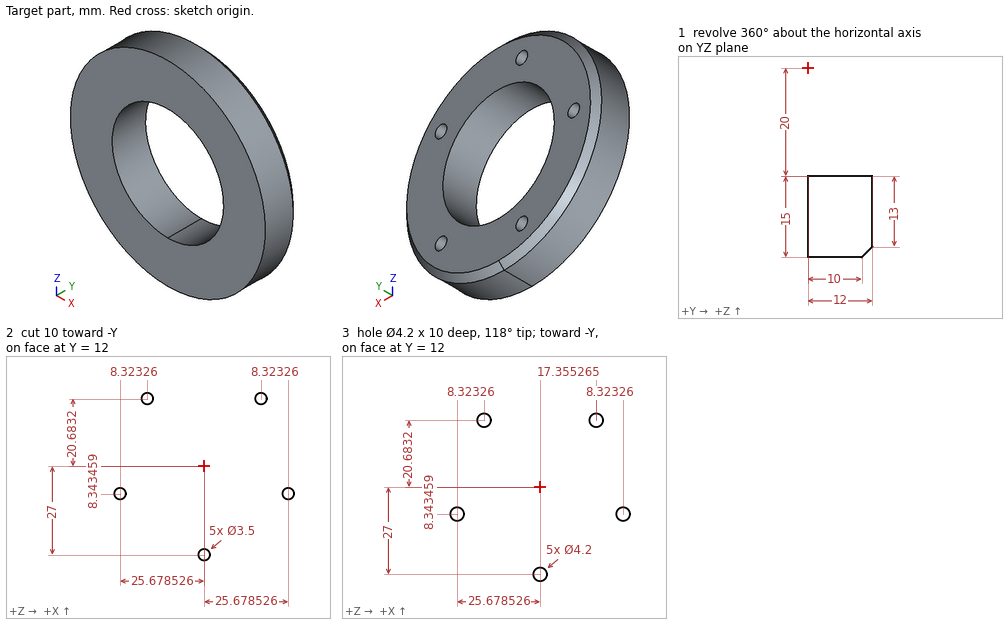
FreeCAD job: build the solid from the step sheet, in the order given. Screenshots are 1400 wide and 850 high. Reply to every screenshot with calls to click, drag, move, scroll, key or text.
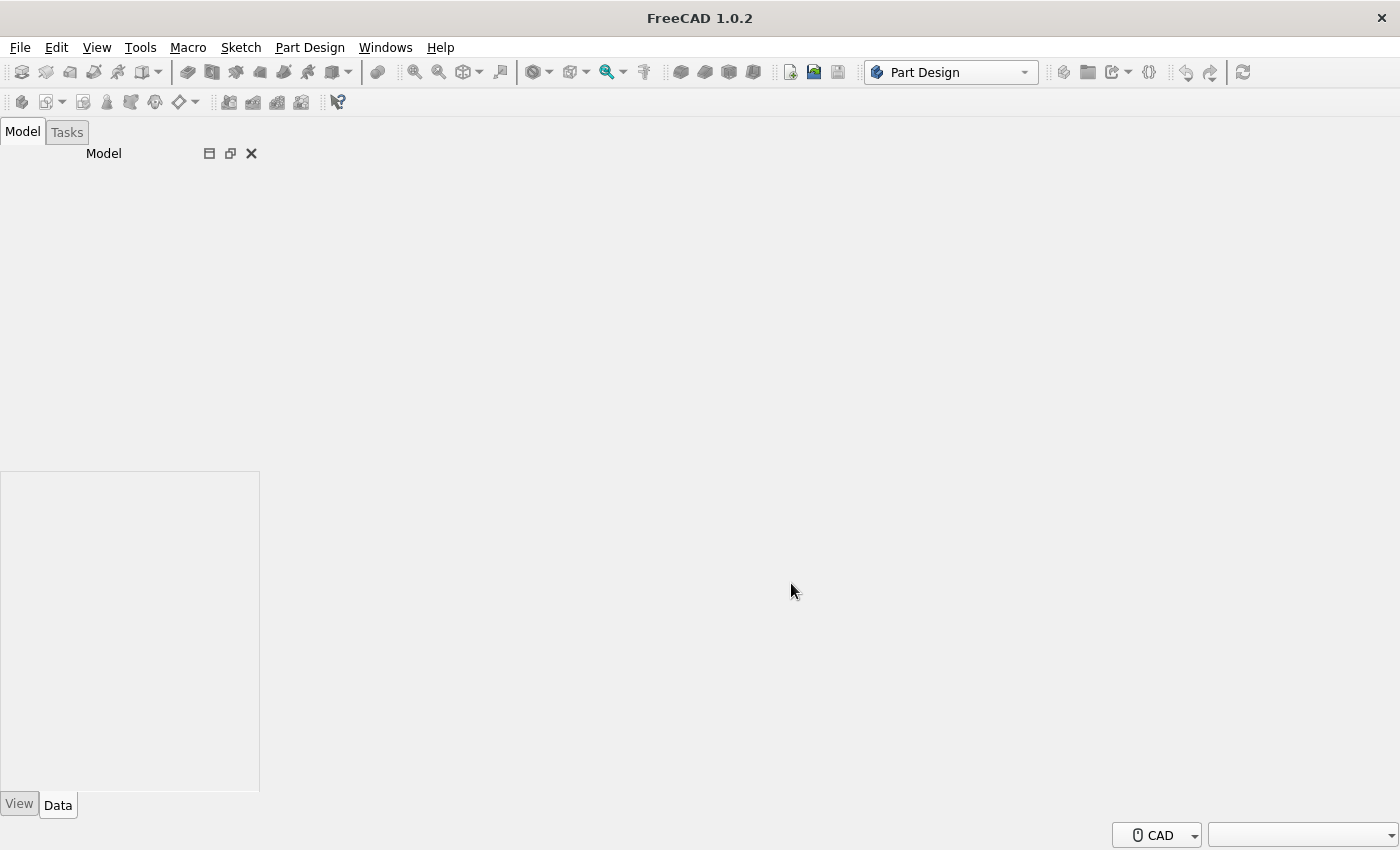
click(790, 72)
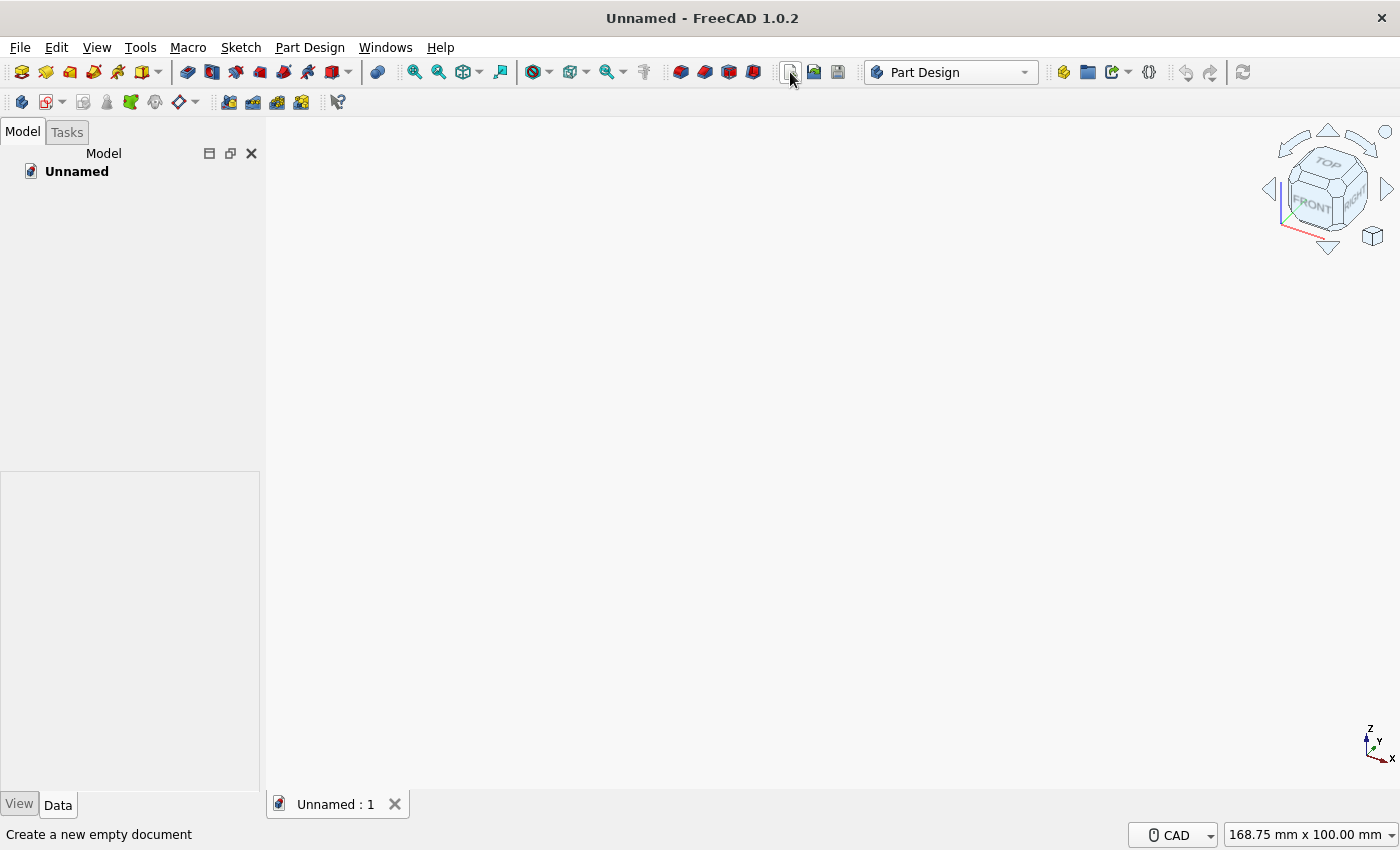
click(46, 102)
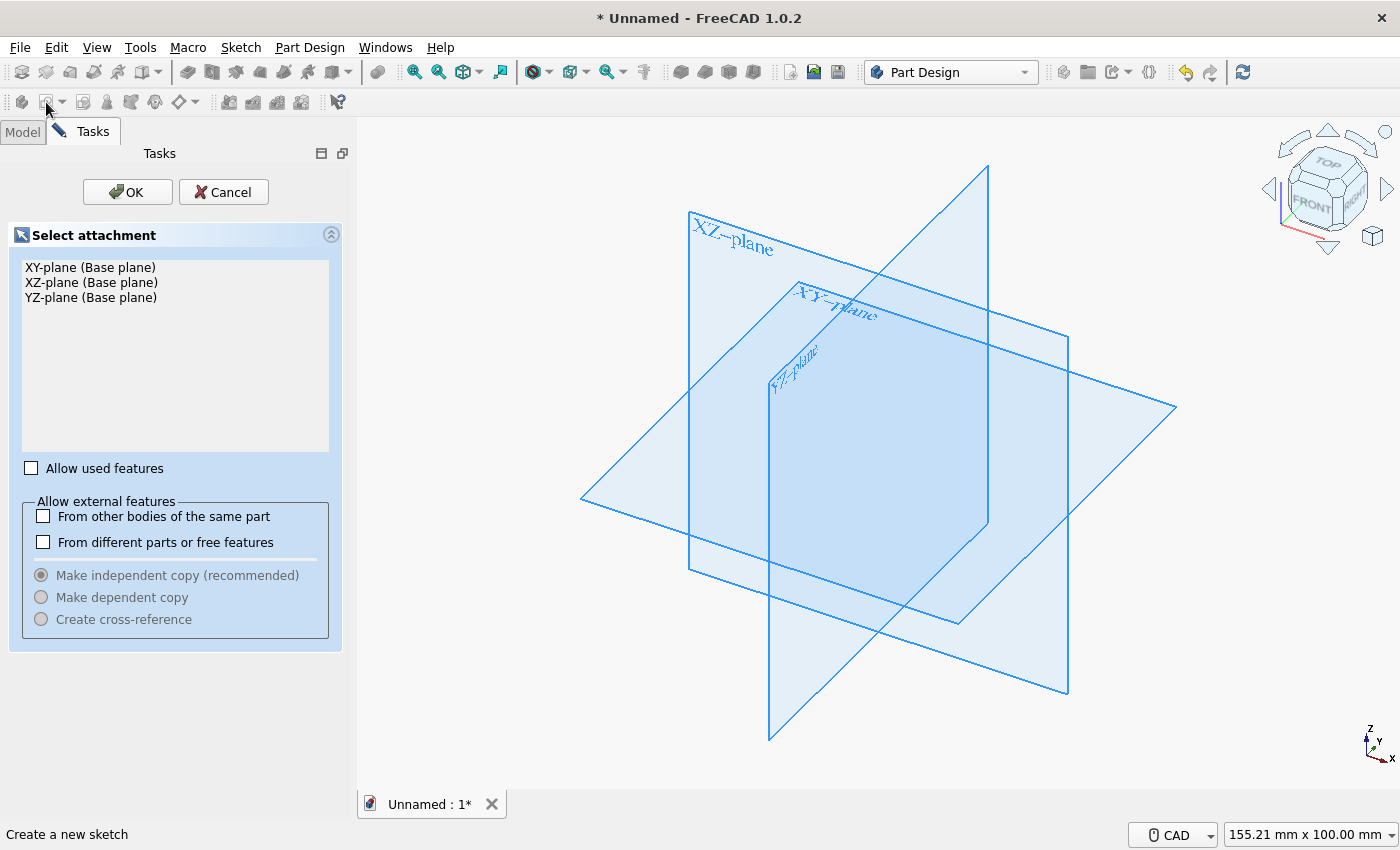
click(82, 298)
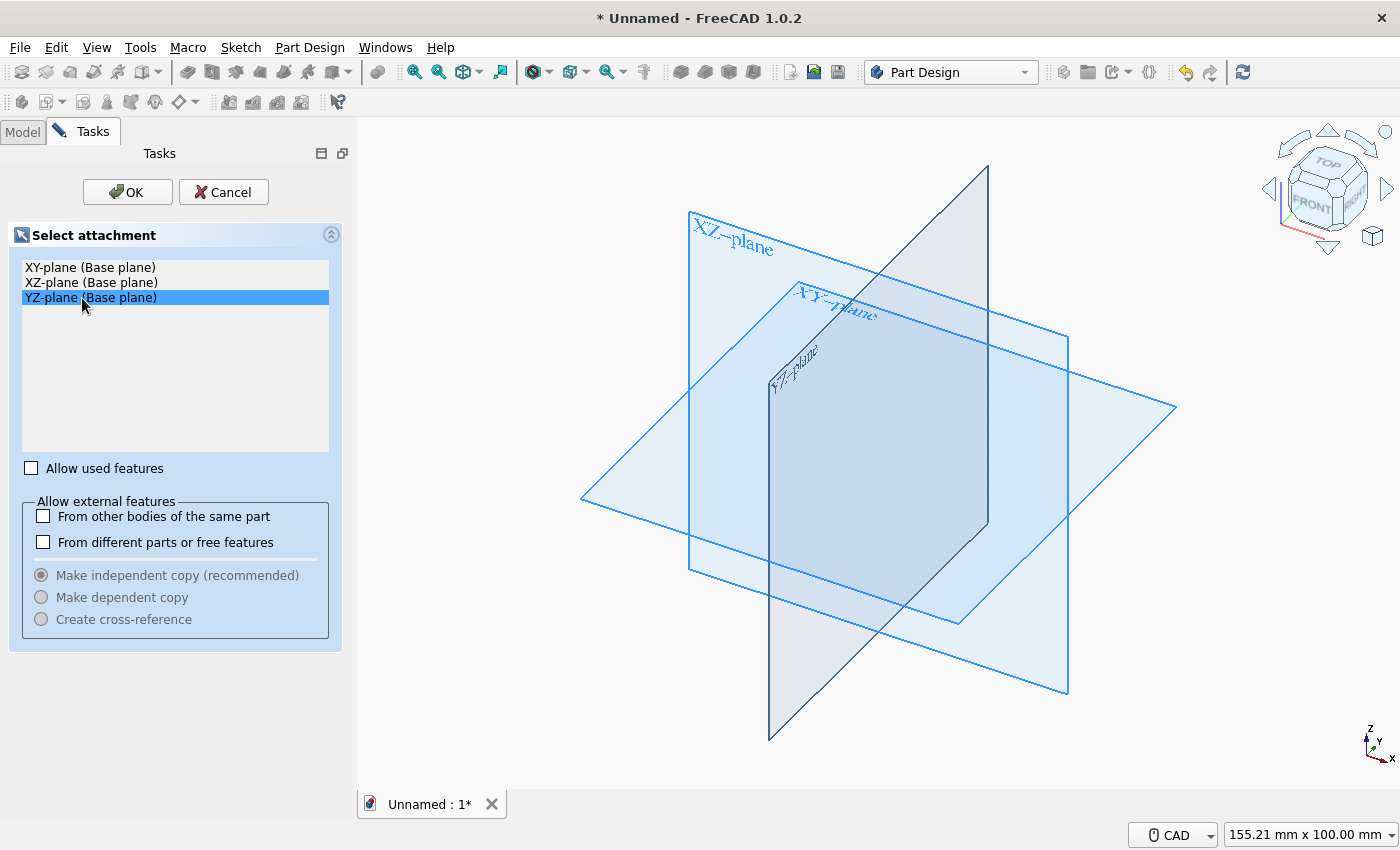
click(128, 192)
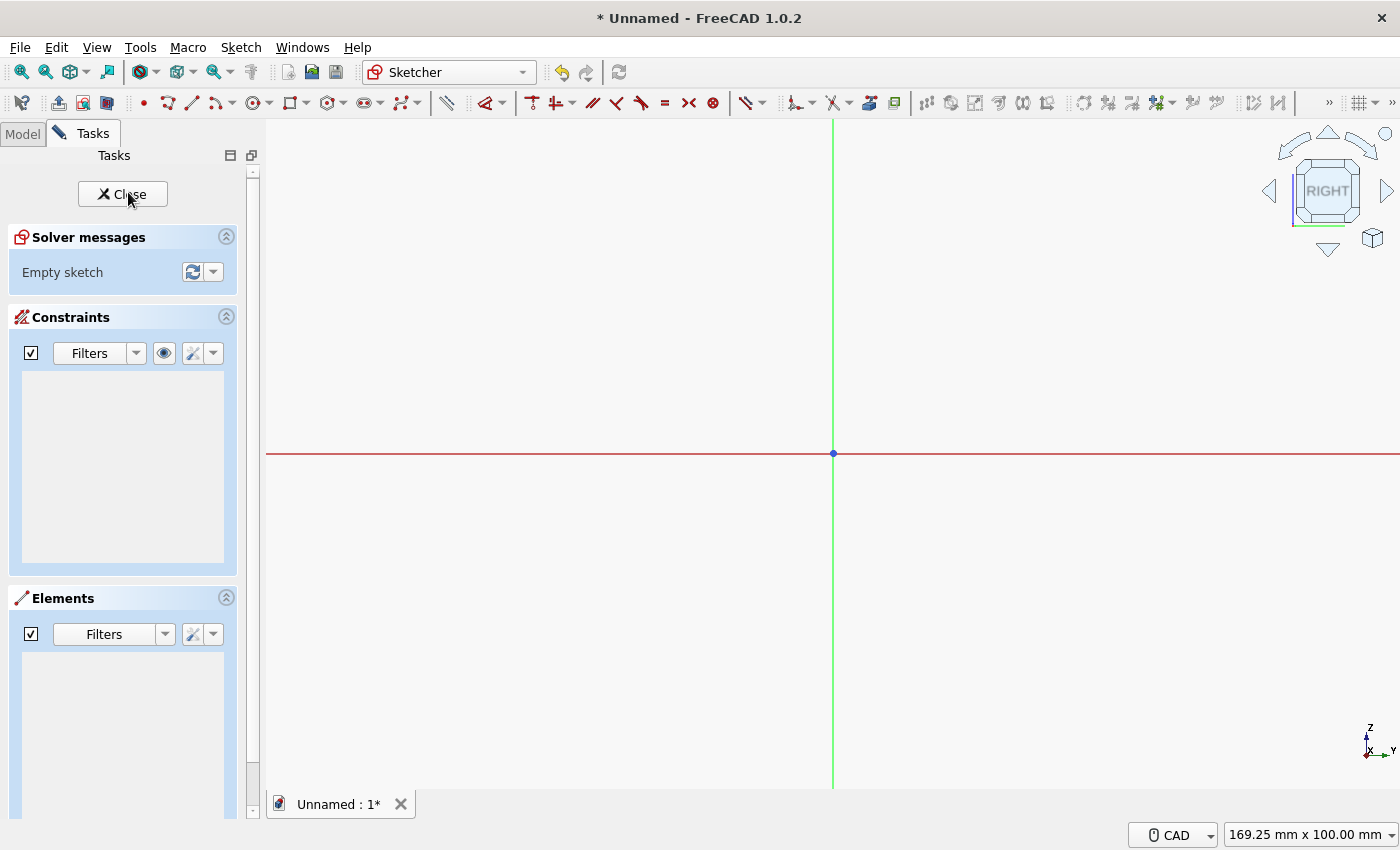
scroll(1005, 714, up, 3)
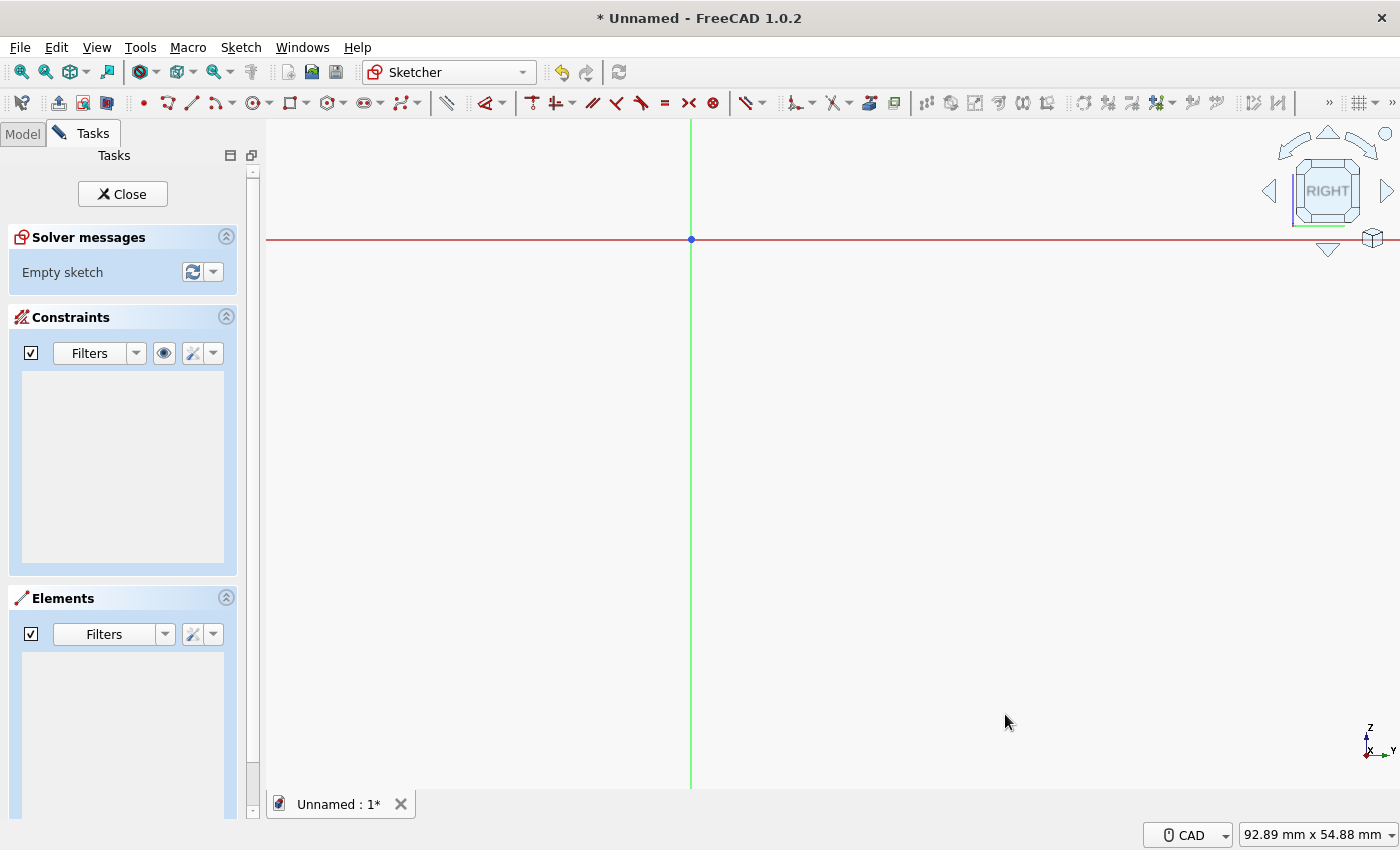
key(g)
key(m)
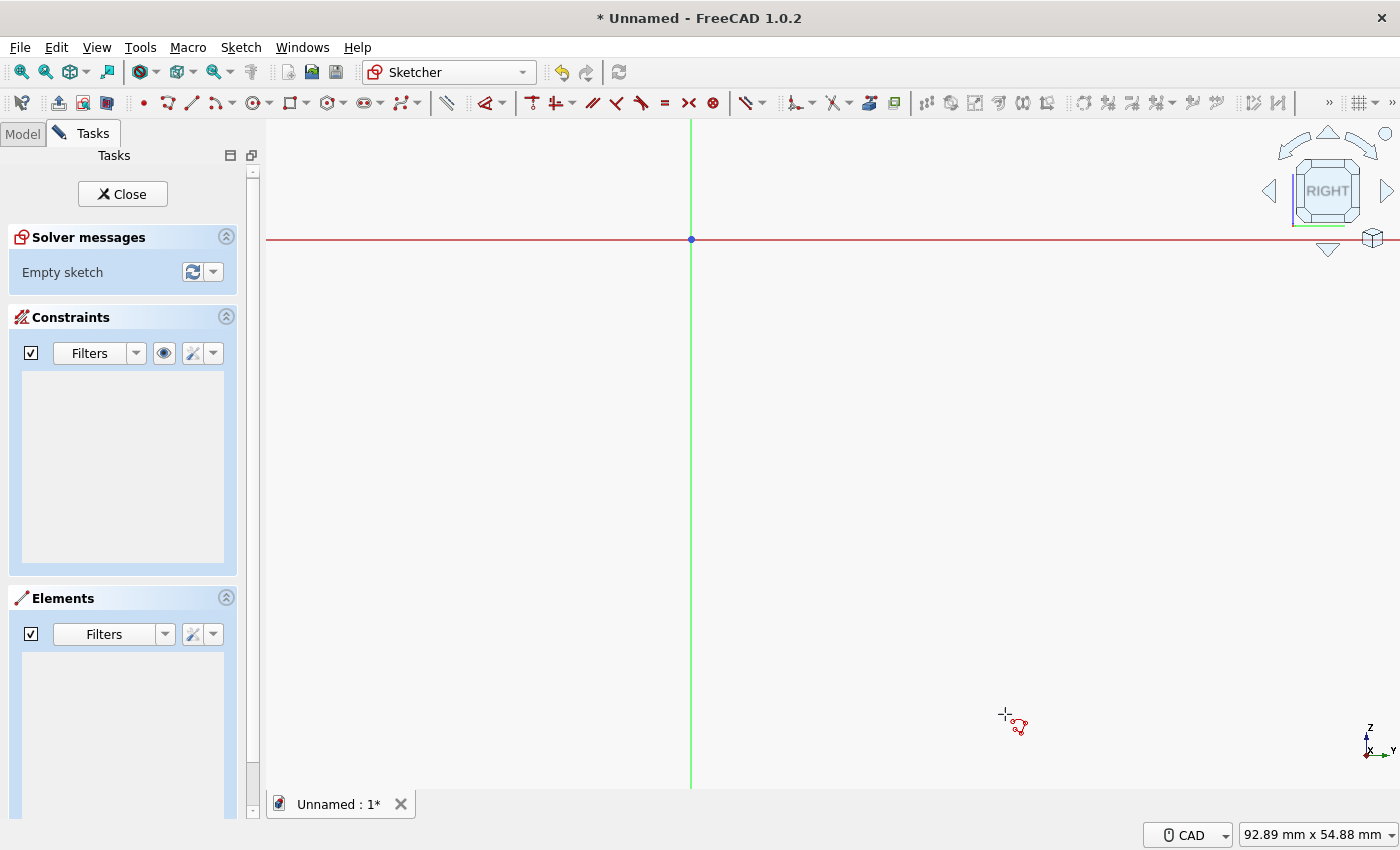
click(691, 484)
click(700, 667)
click(813, 667)
click(838, 642)
click(838, 484)
click(691, 485)
key(Escape)
key(Escape)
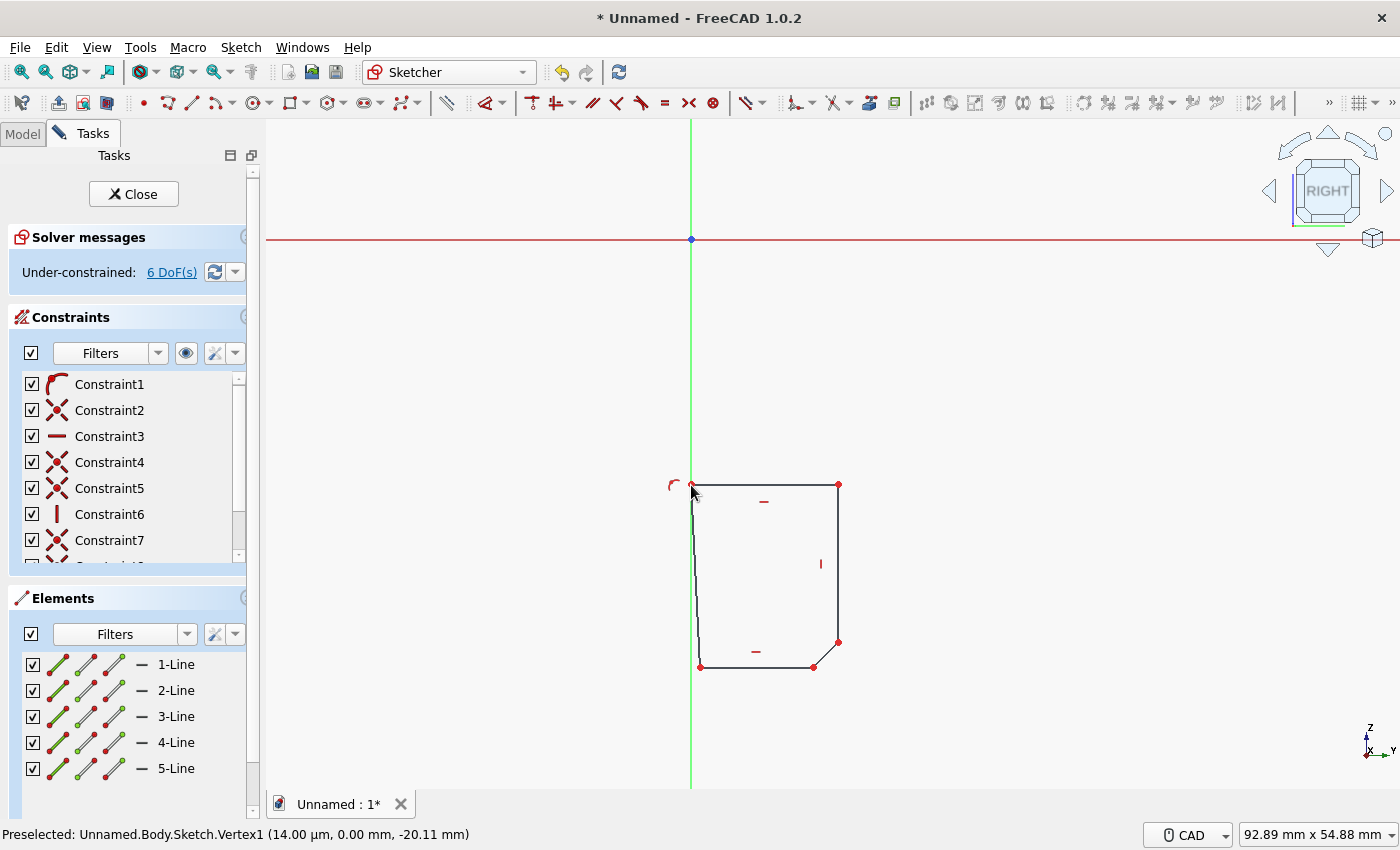
click(694, 540)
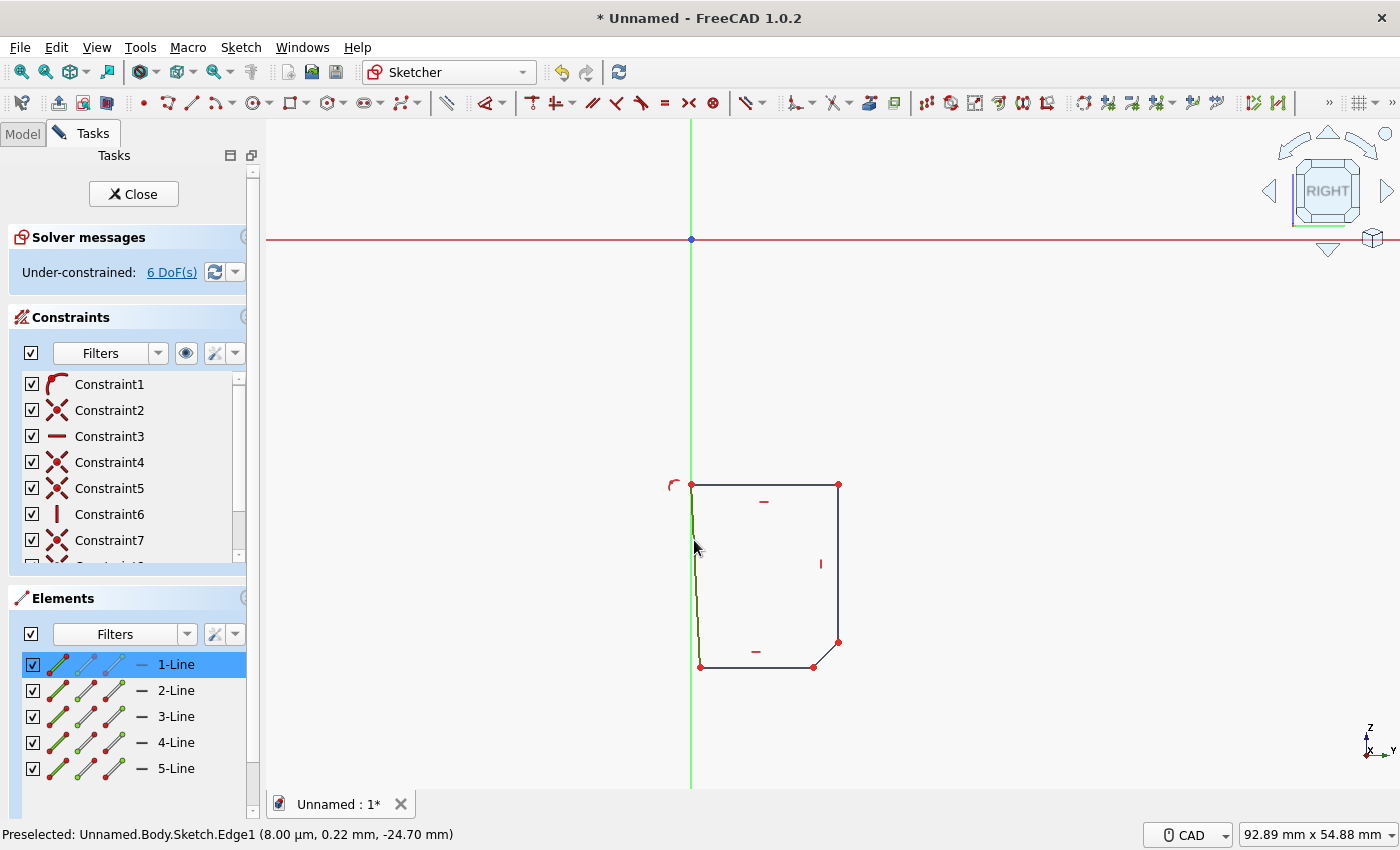
key(v)